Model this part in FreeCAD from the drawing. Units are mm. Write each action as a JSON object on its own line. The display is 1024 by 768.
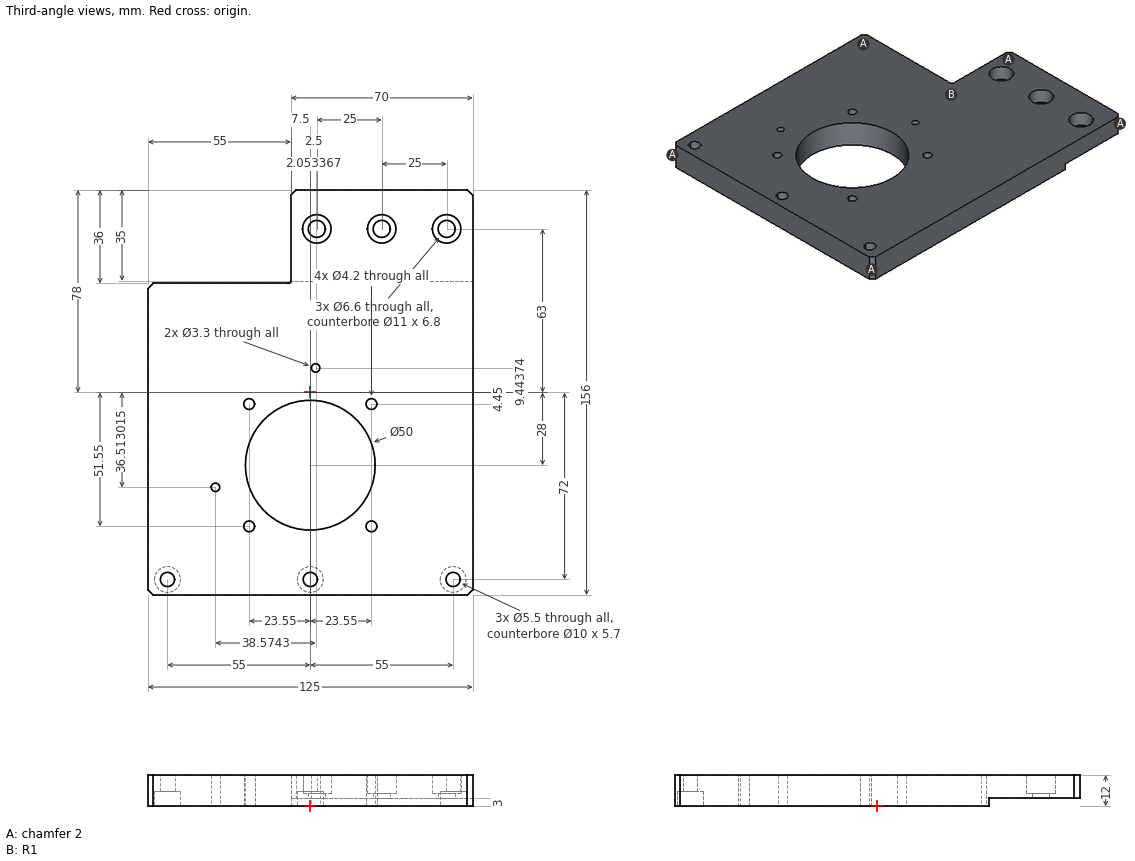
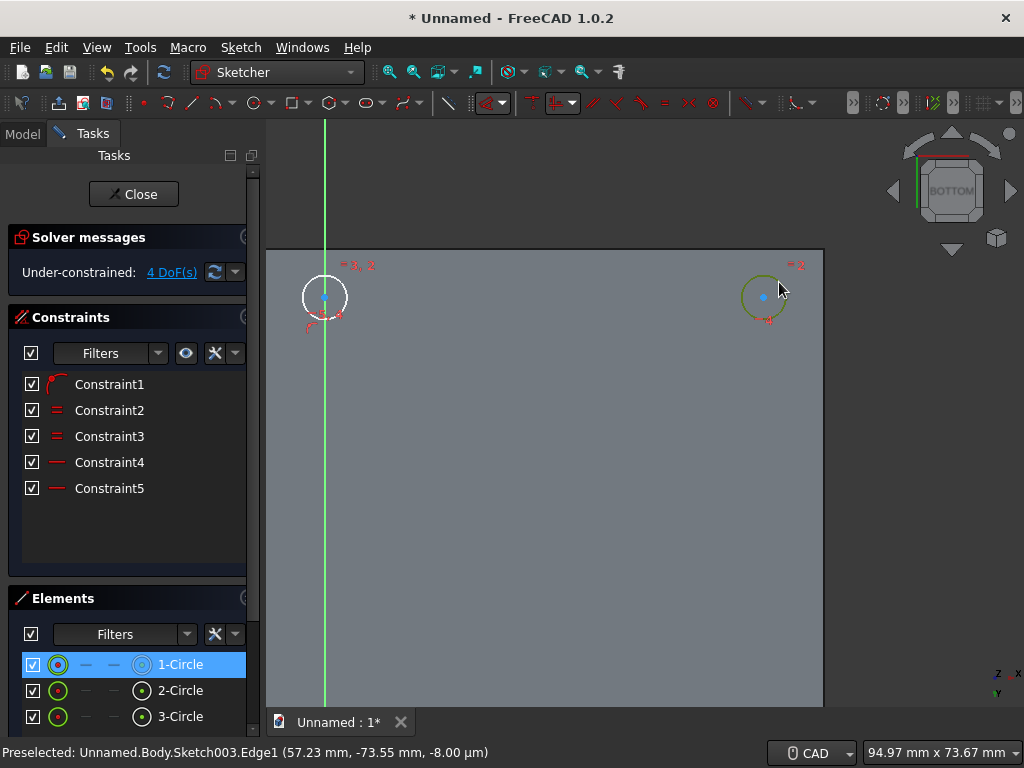
{"action": "key", "text": "k o"}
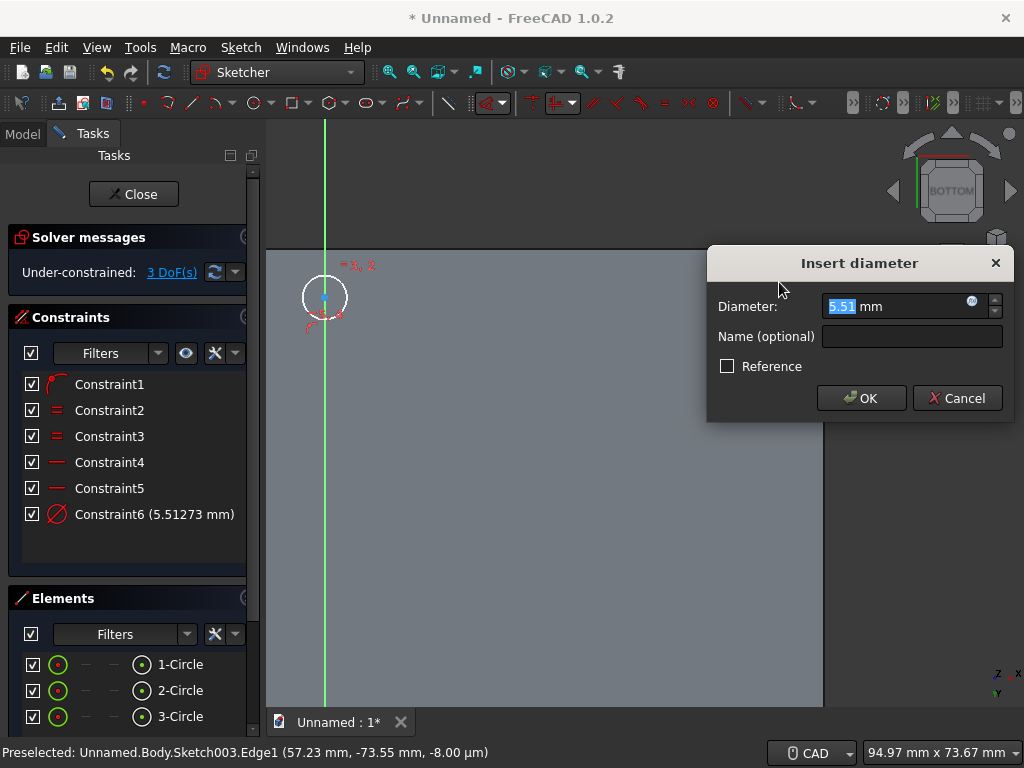
{"action": "type", "text": "5.5"}
{"action": "key", "text": "Return"}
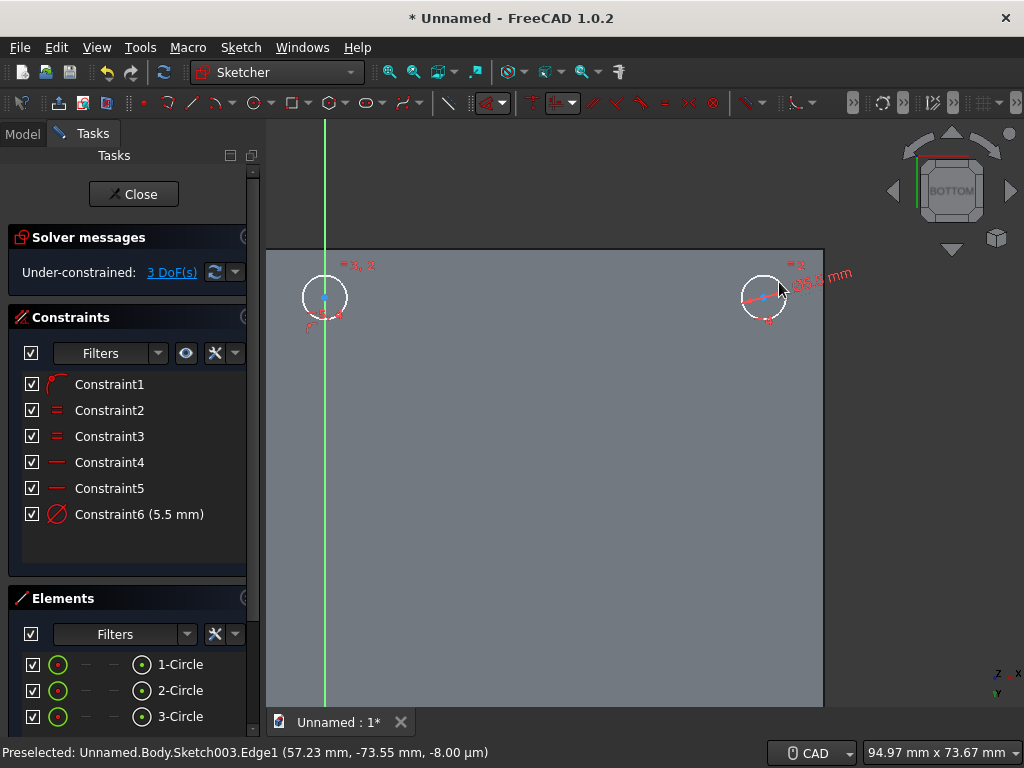
{"action": "left_click", "coordinate": [764, 297]}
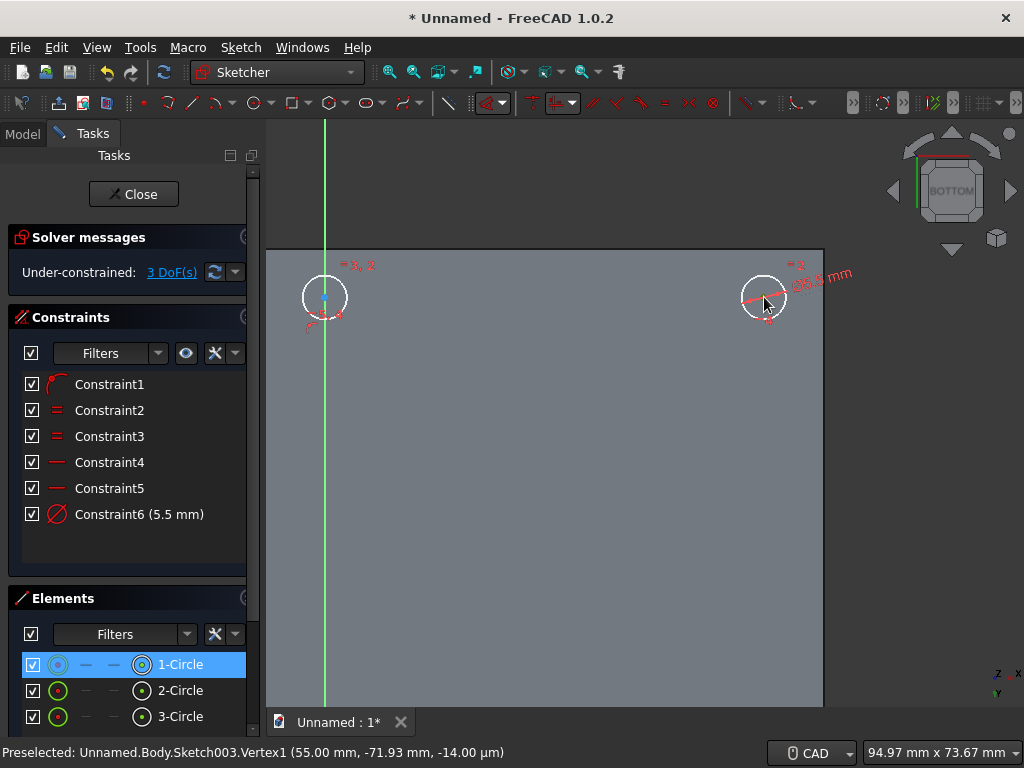
{"action": "left_click", "coordinate": [504, 104]}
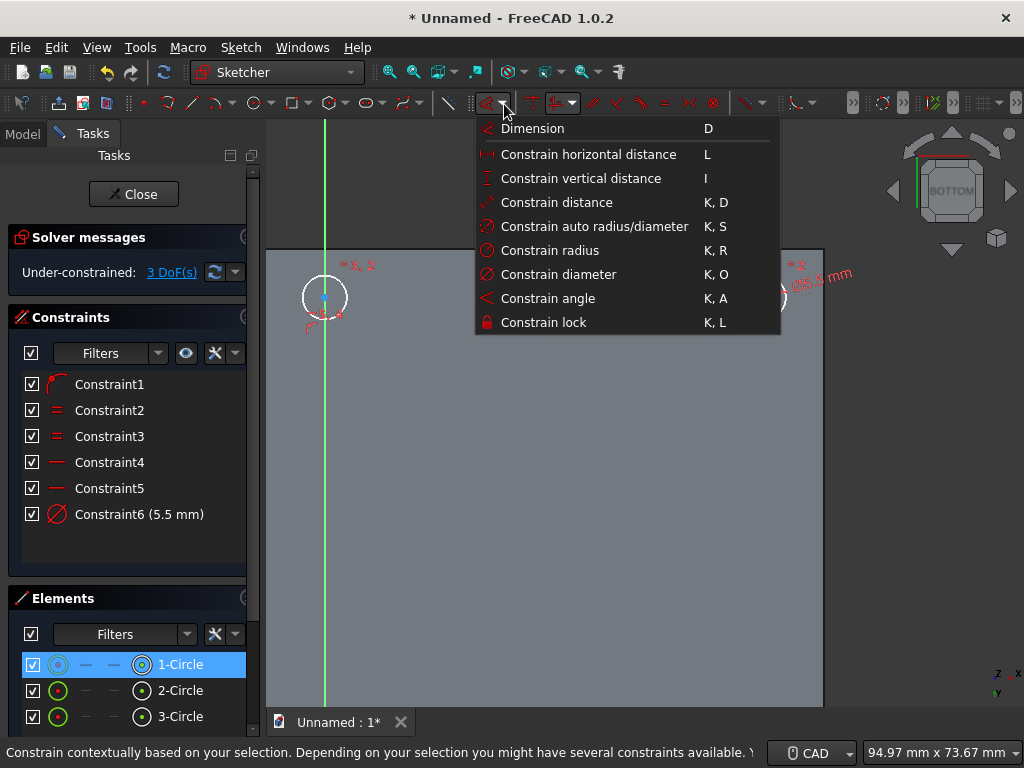
{"action": "left_click", "coordinate": [628, 154]}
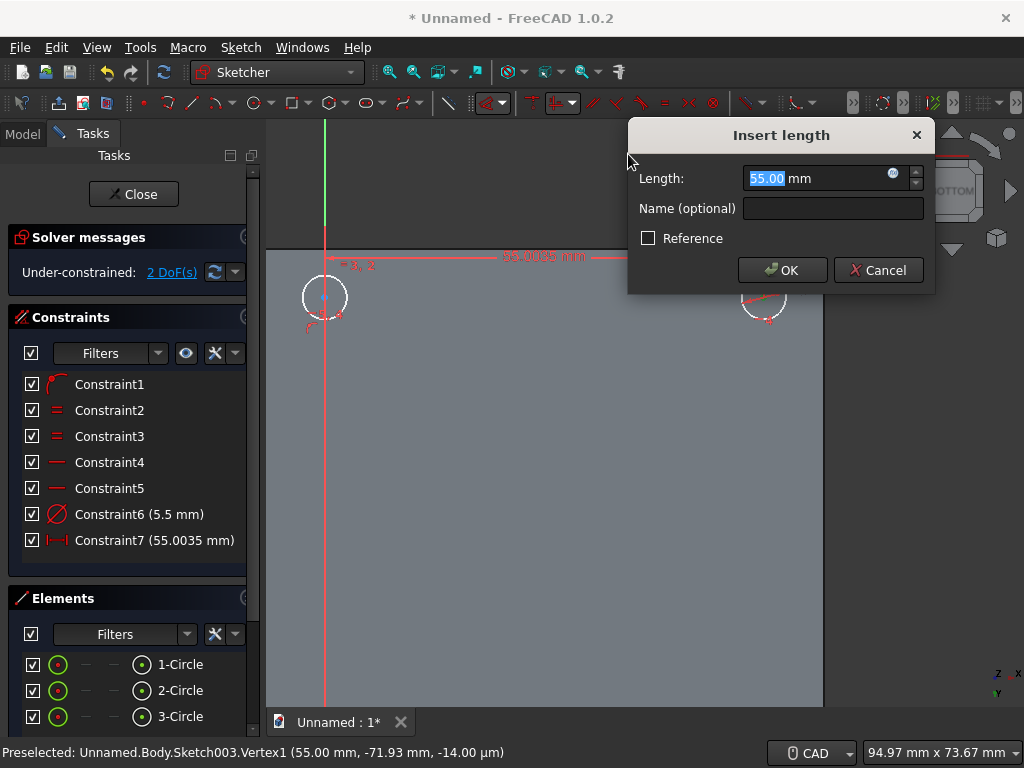
{"action": "type", "text": "55"}
{"action": "key", "text": "Return"}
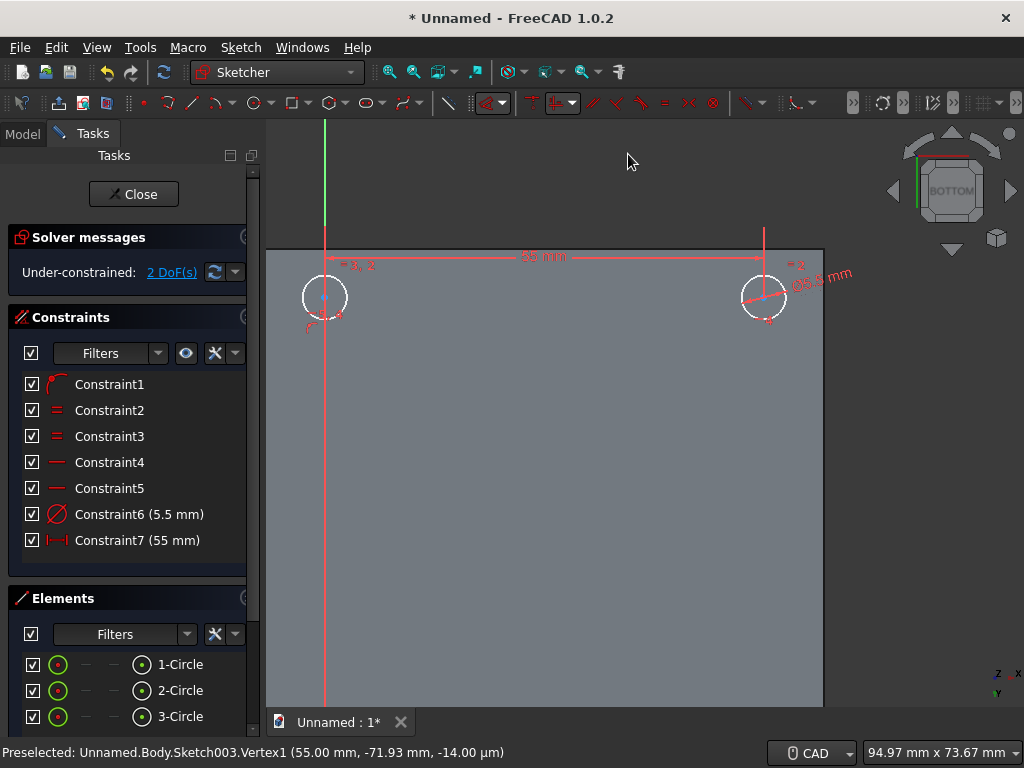
{"action": "left_click", "coordinate": [764, 297]}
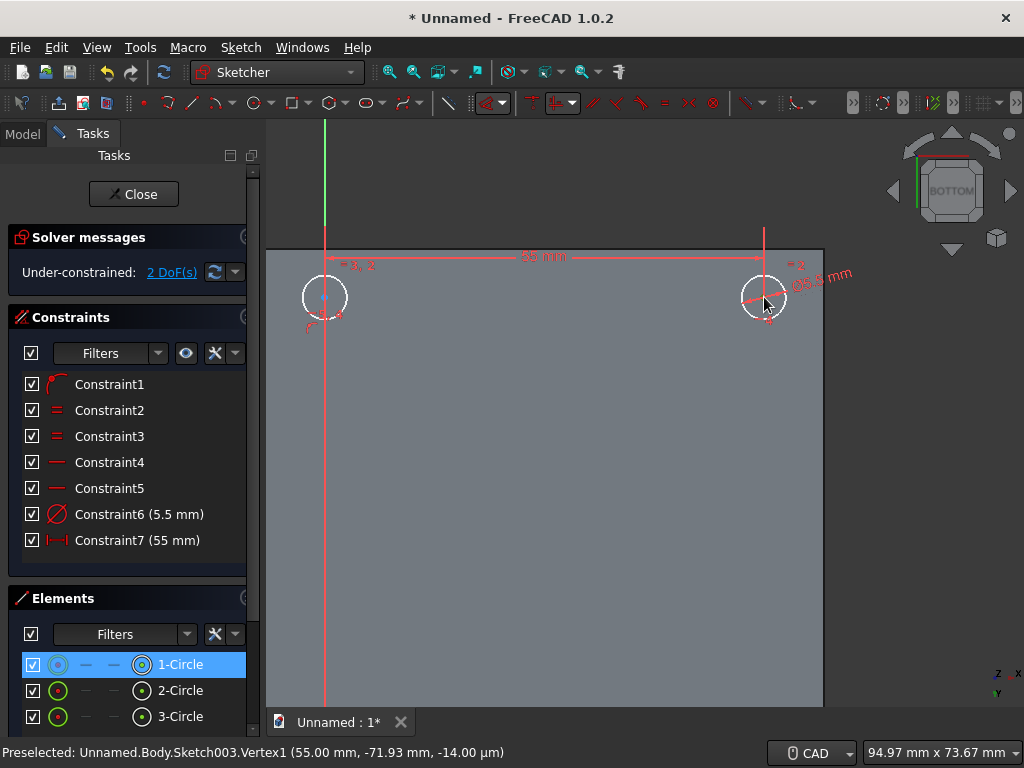
{"action": "key", "text": "i"}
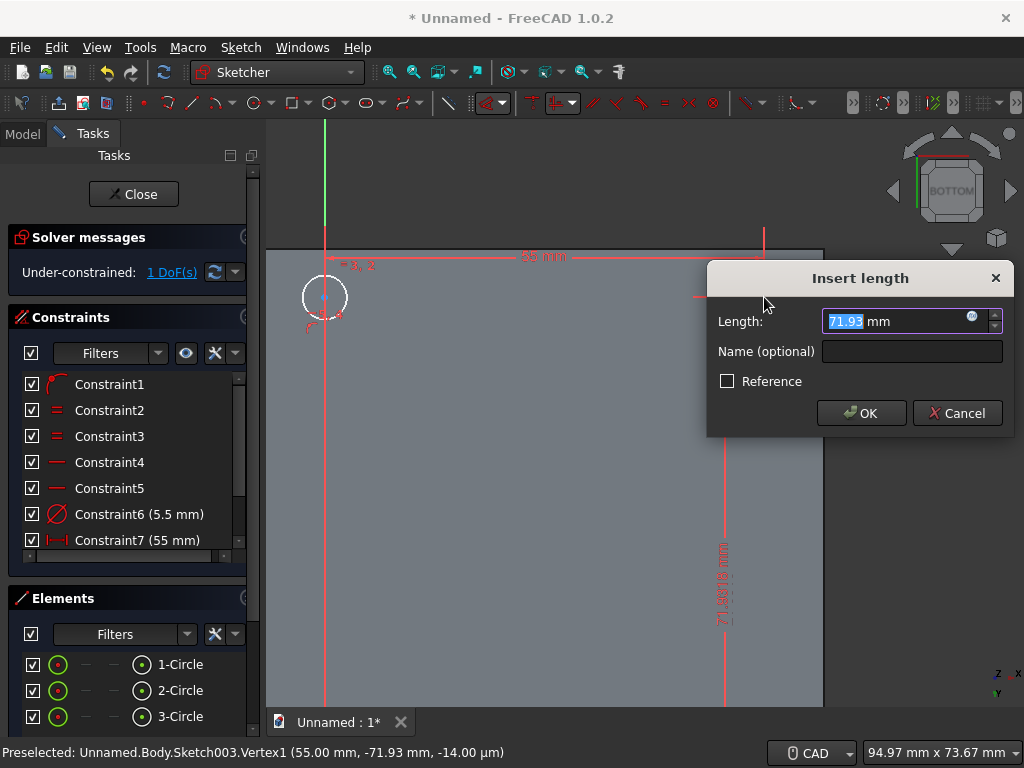
{"action": "type", "text": "72"}
{"action": "key", "text": "Return"}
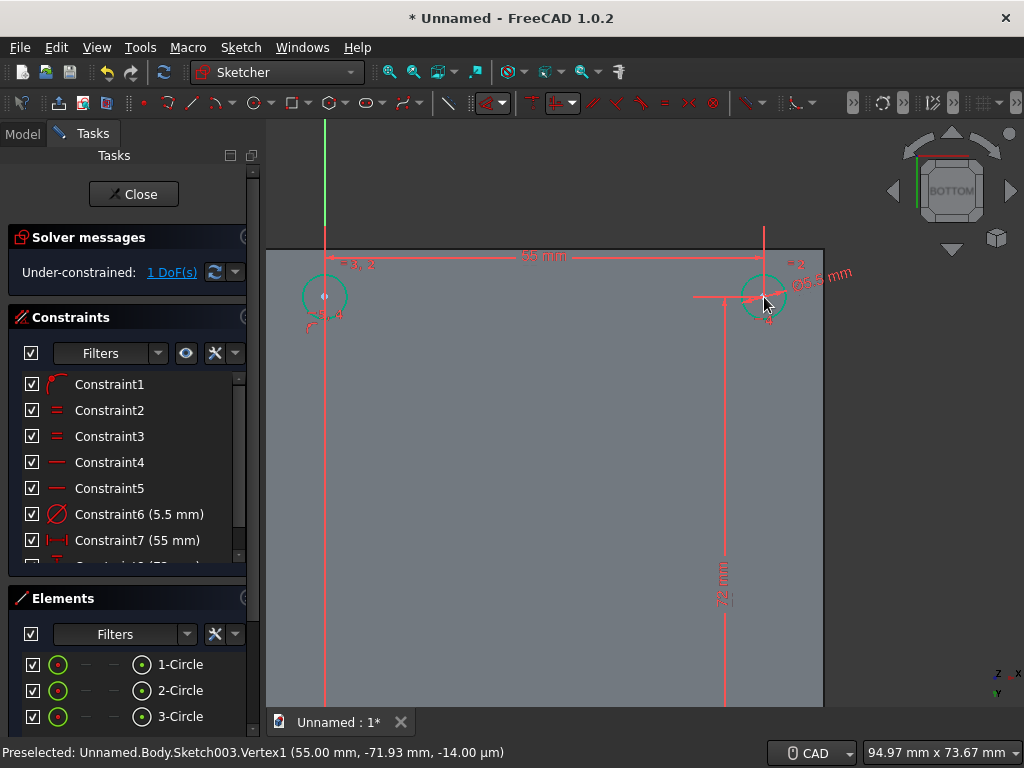
{"action": "scroll", "coordinate": [782, 282], "scroll_direction": "down", "scroll_amount": 4}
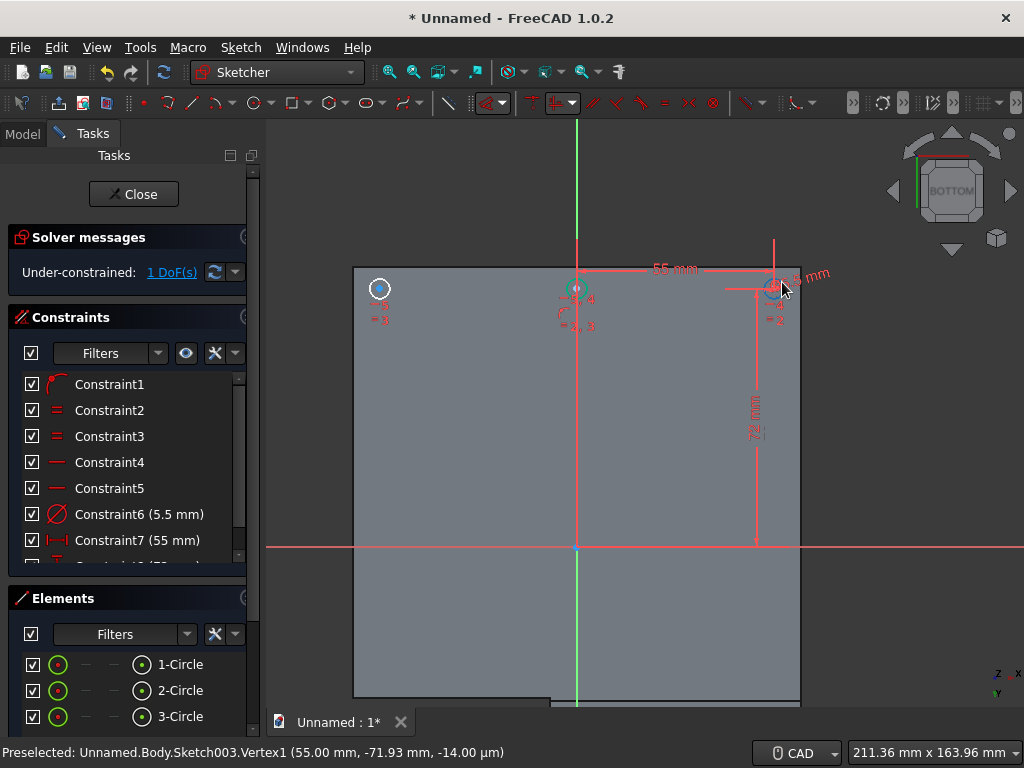
{"action": "left_click", "coordinate": [380, 289]}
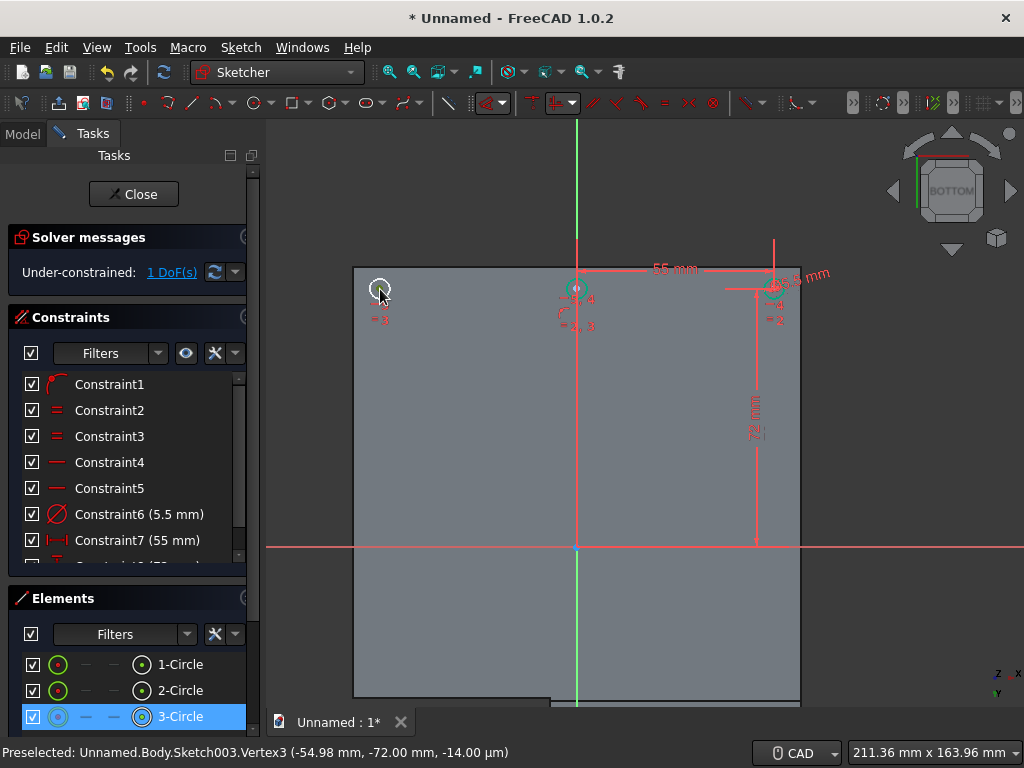
{"action": "left_click", "coordinate": [504, 104]}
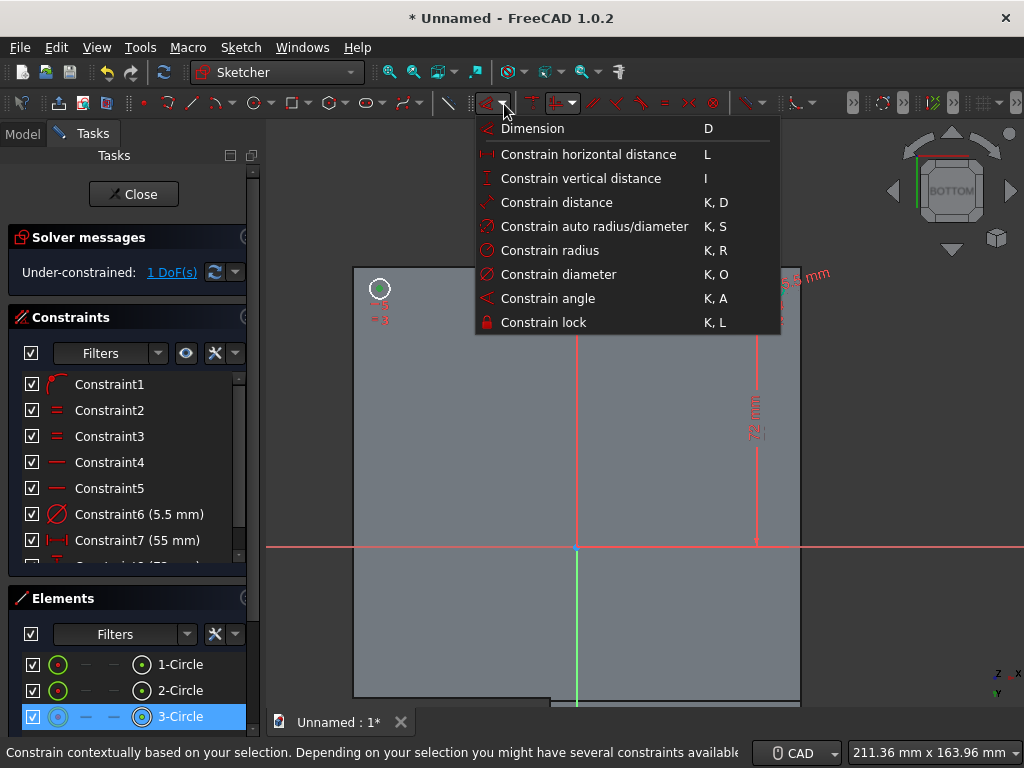
{"action": "left_click", "coordinate": [628, 154]}